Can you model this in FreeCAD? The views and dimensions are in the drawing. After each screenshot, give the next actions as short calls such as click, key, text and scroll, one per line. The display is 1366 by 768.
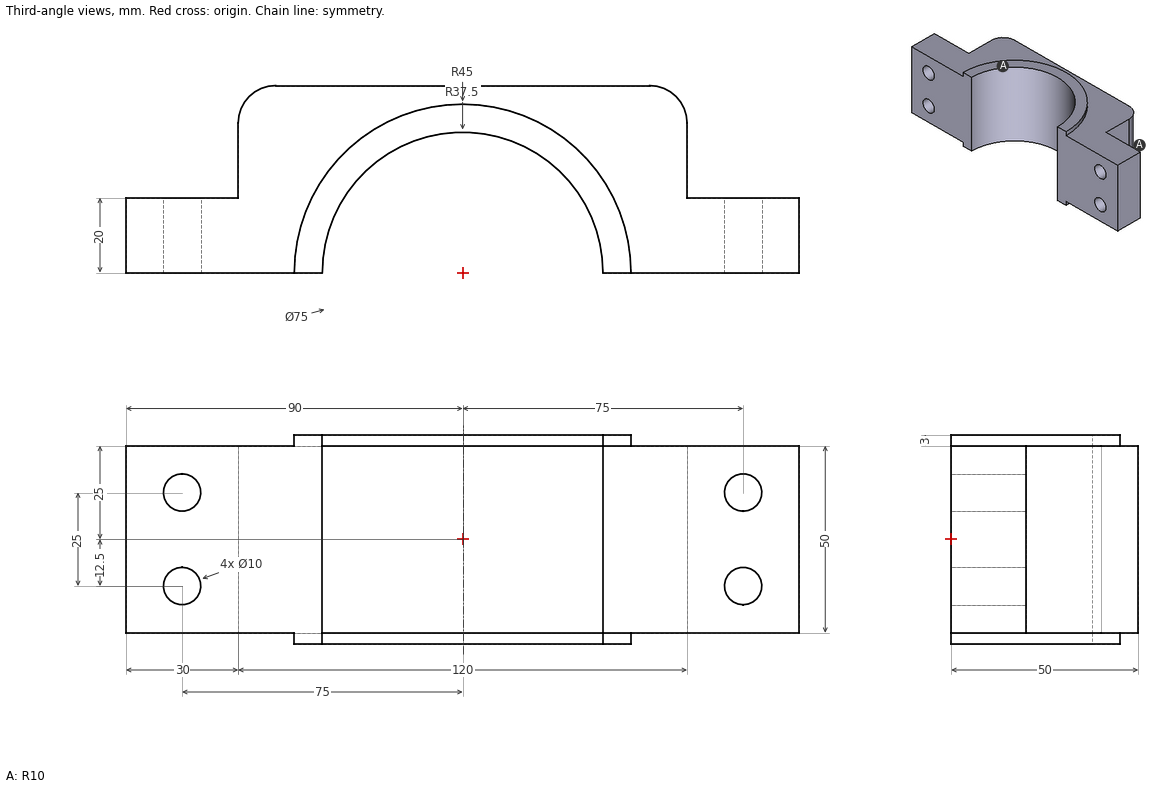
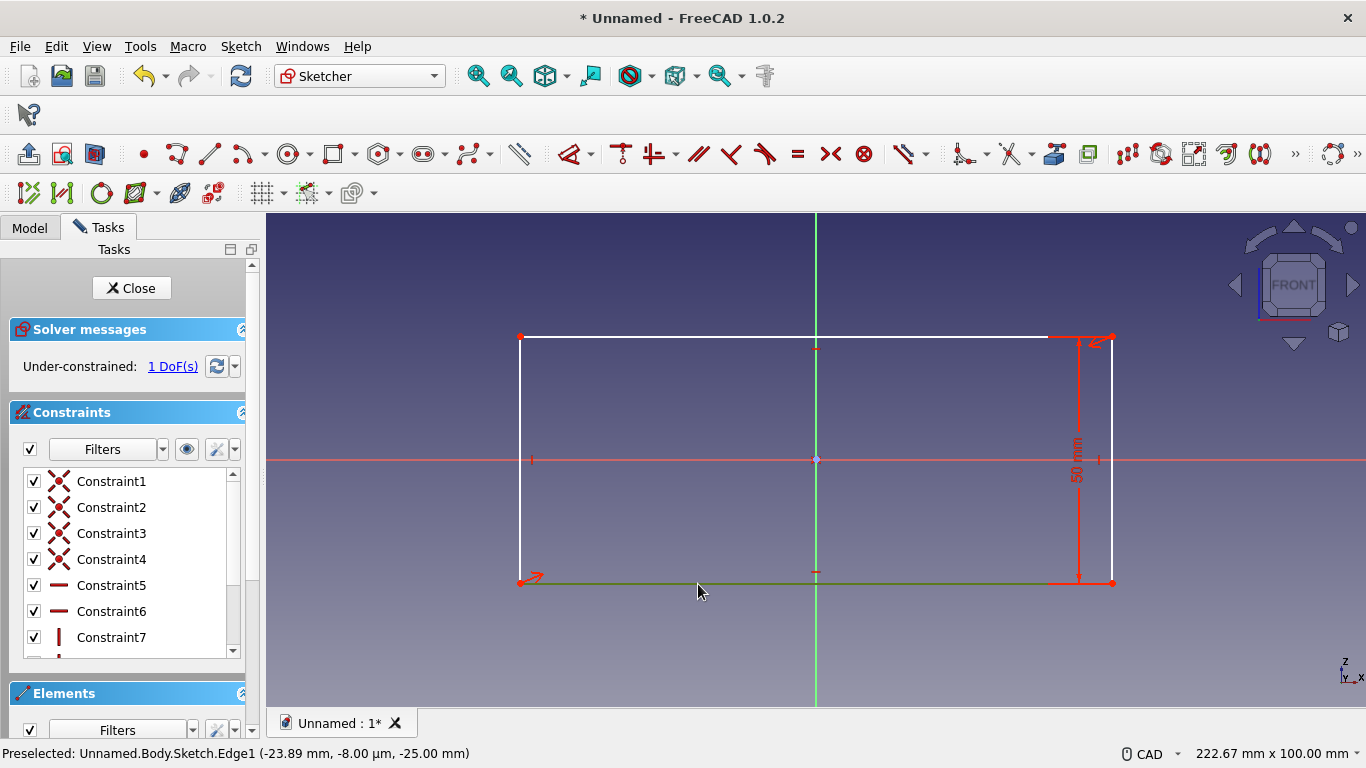
key(l)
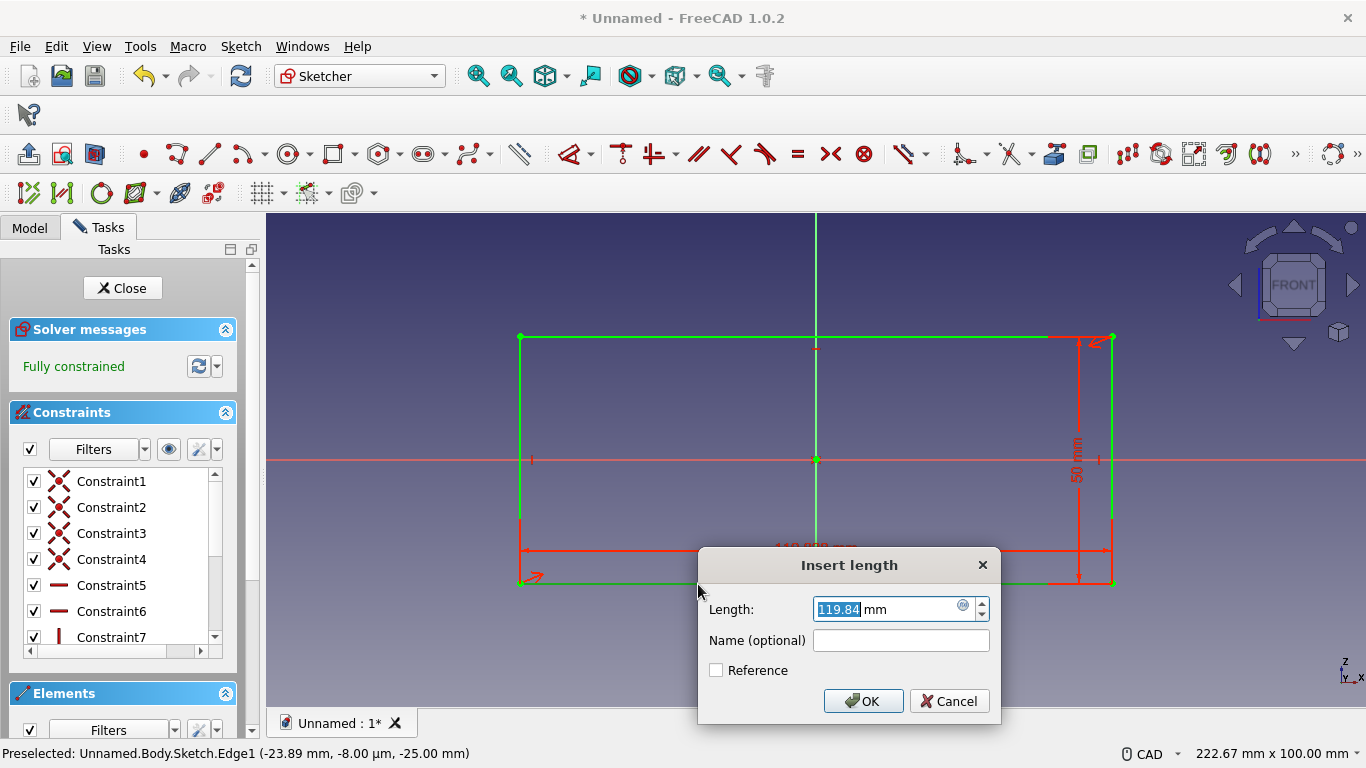
text(120)
key(Return)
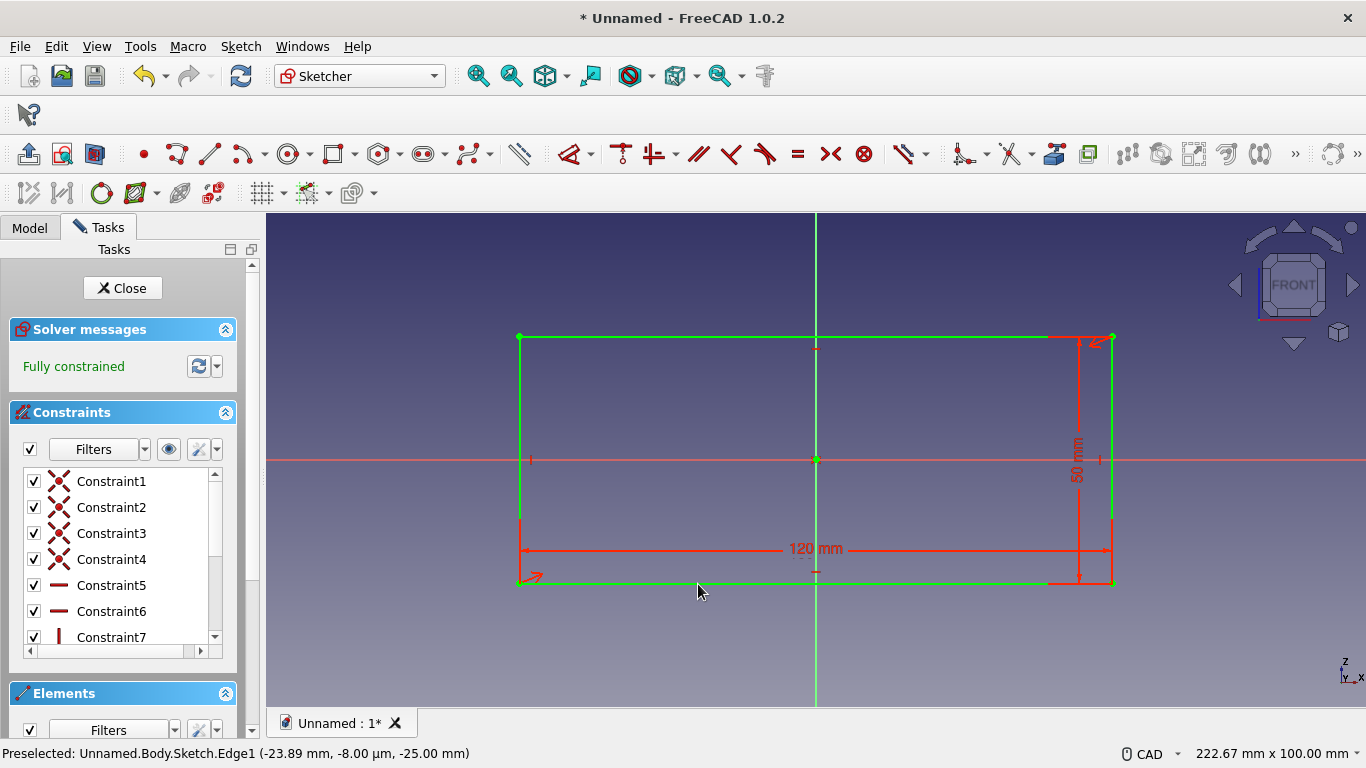
click(123, 288)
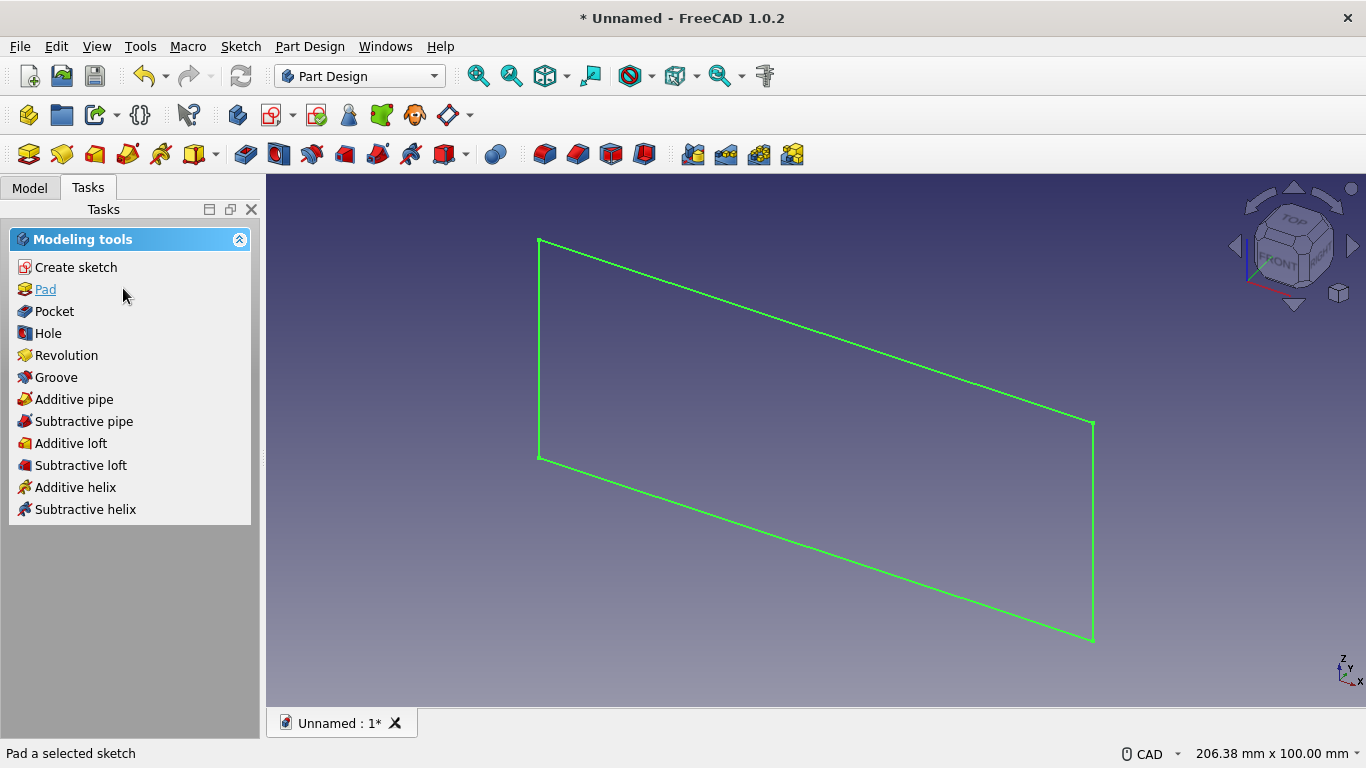
click(29, 154)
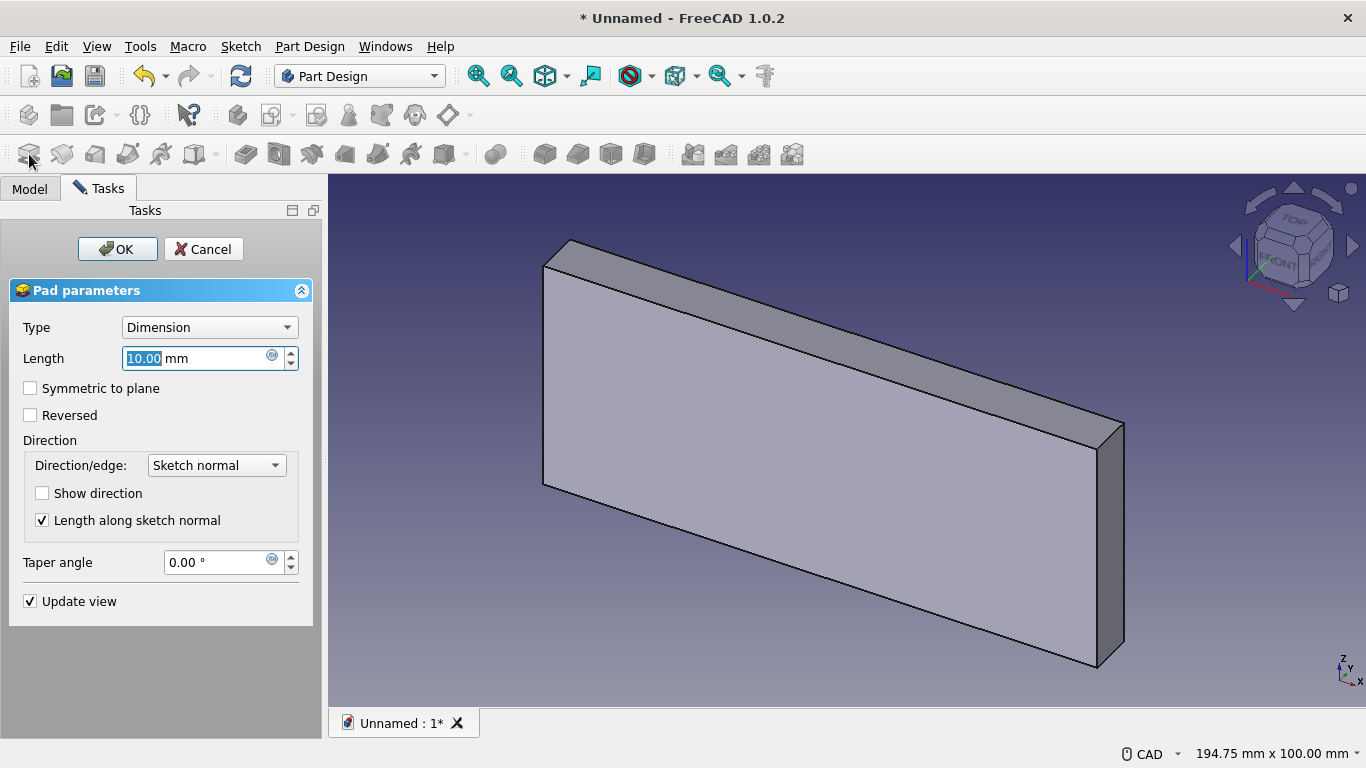
text(50)
key(Tab)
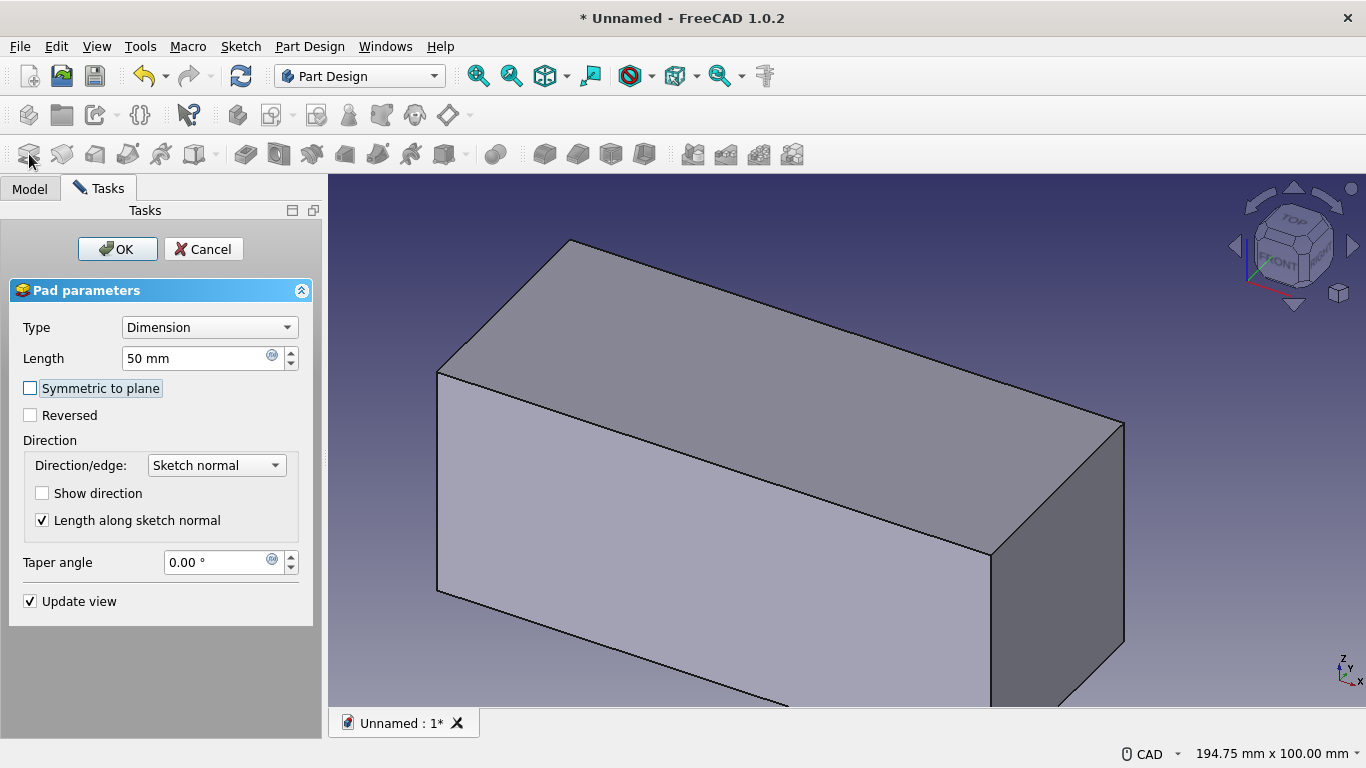
click(31, 415)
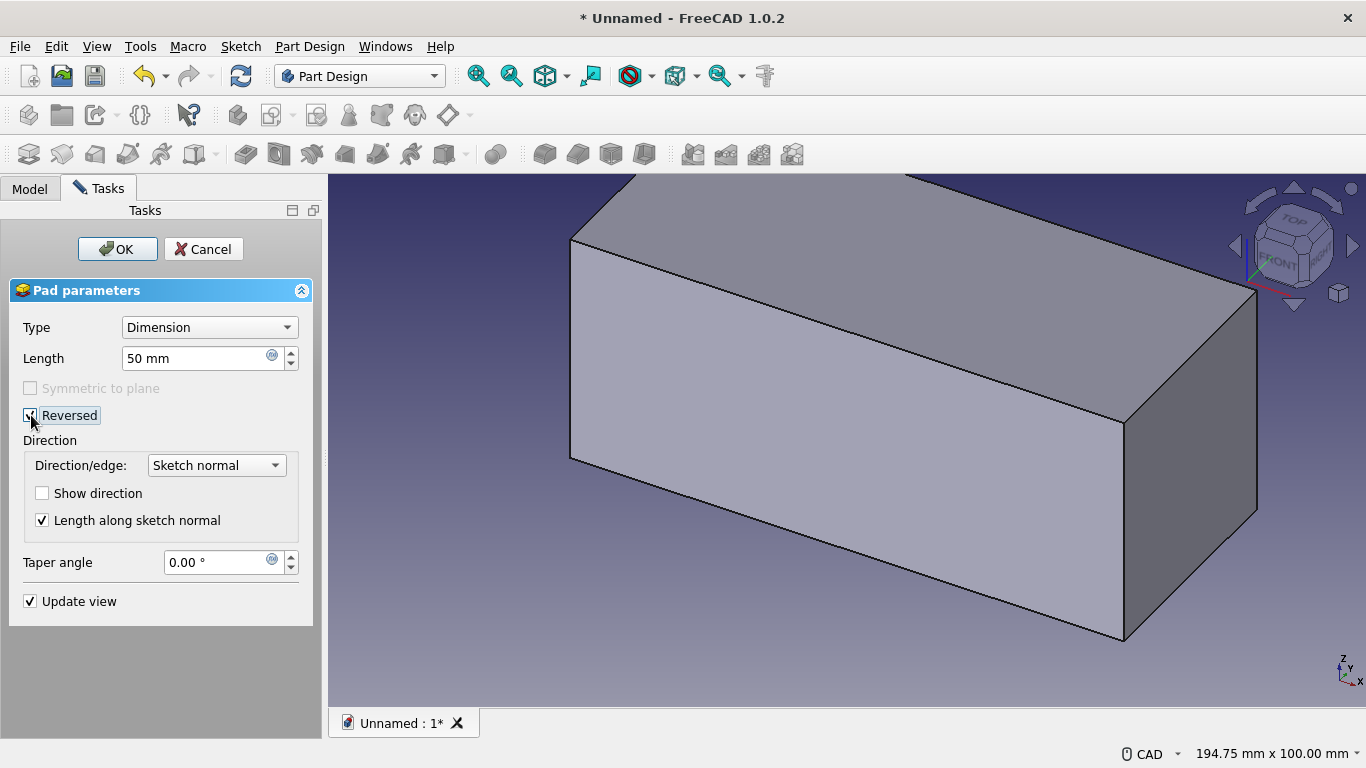
click(118, 249)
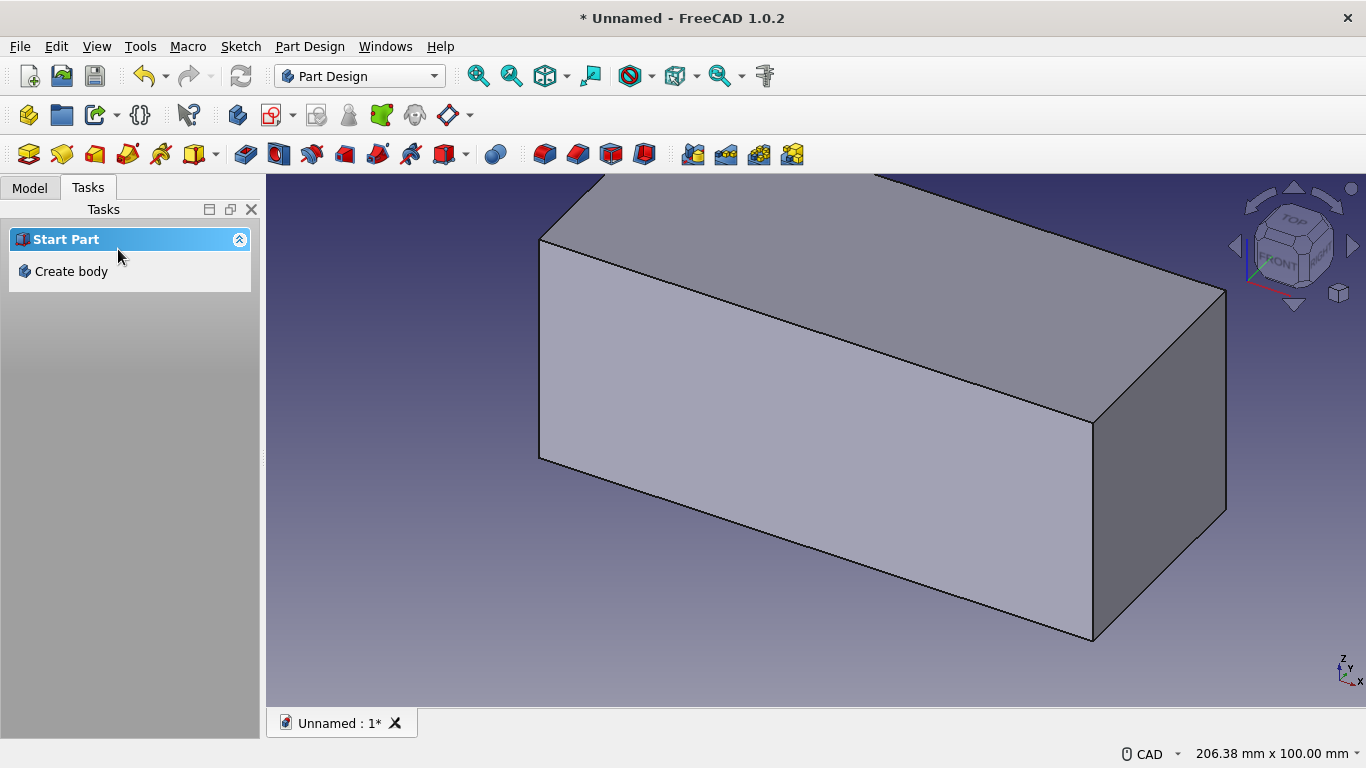
key(v)
key(f)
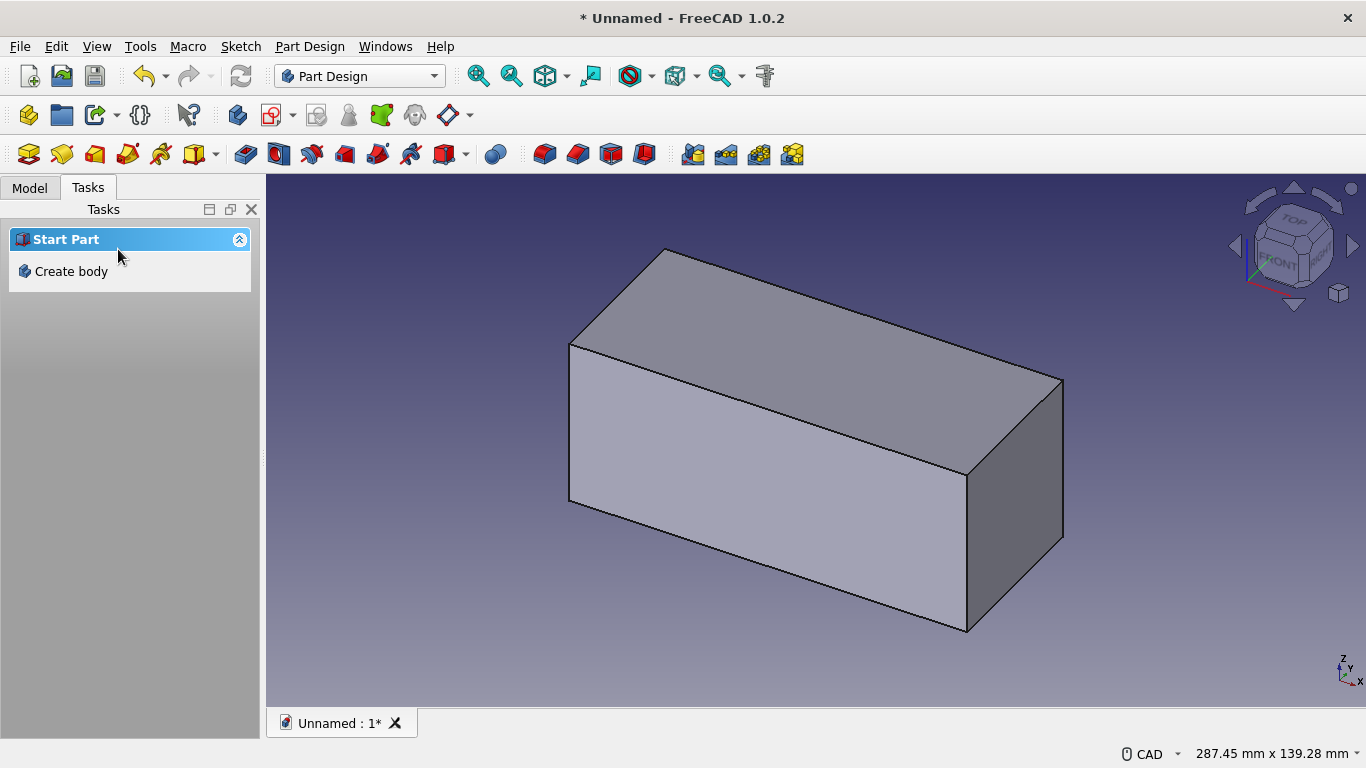
click(930, 399)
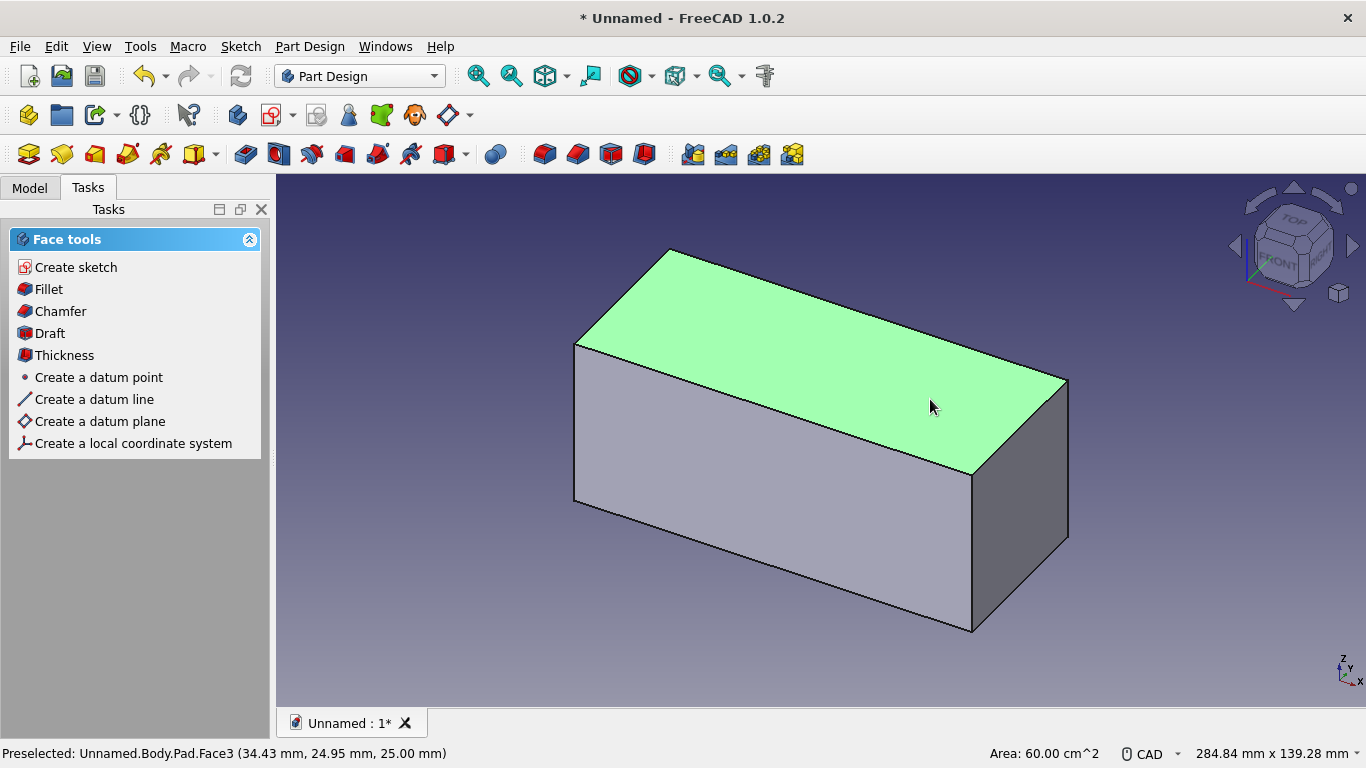
click(270, 116)